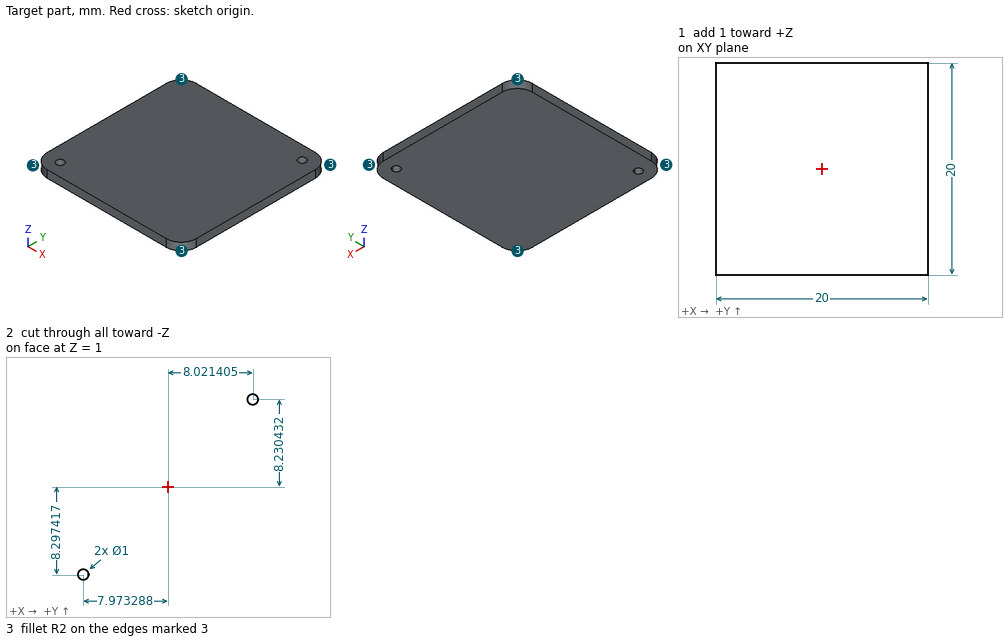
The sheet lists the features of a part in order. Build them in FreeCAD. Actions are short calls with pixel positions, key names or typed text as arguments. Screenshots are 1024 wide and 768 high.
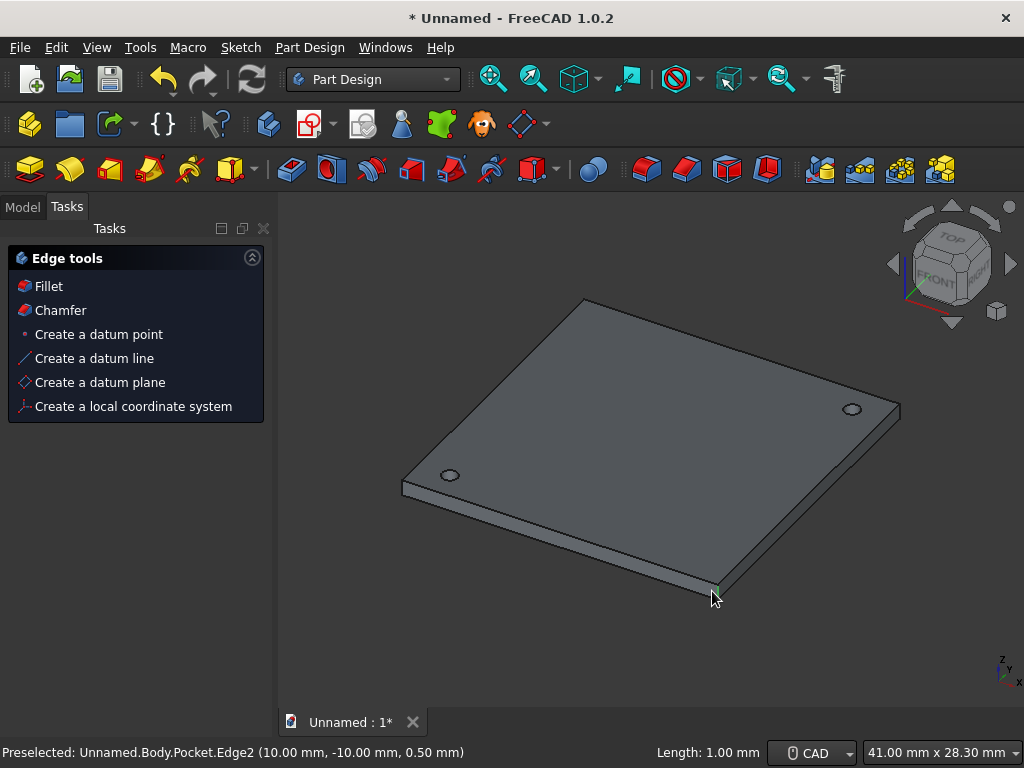
scroll(402, 487, up, 4)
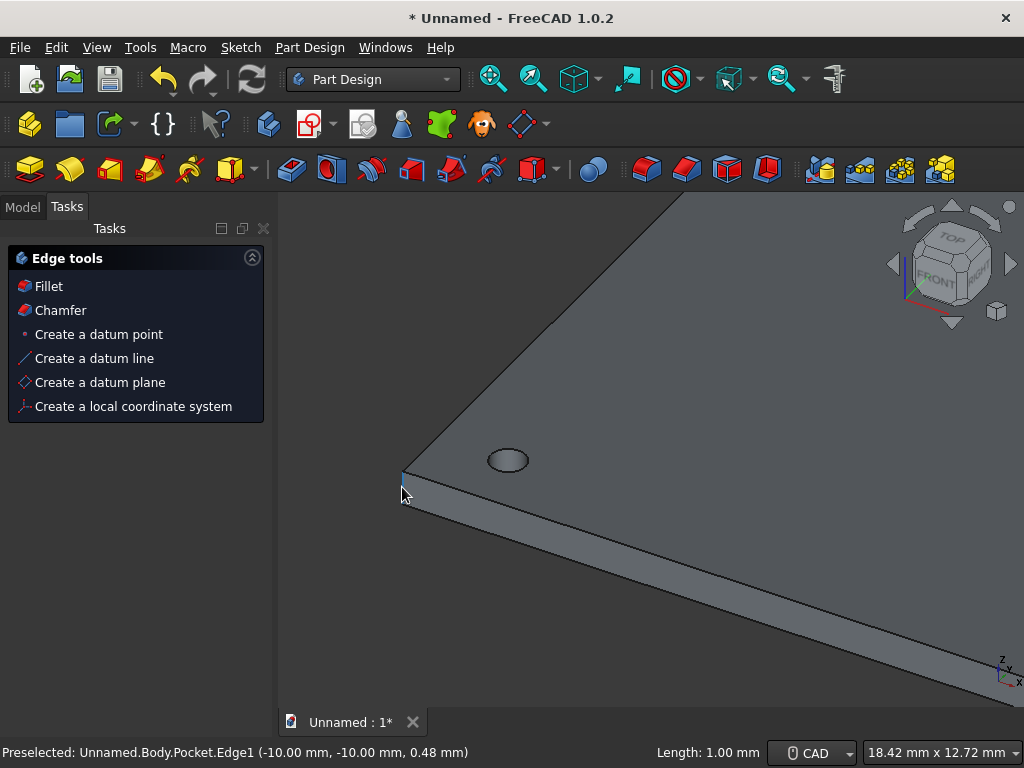
key(v)
key(f)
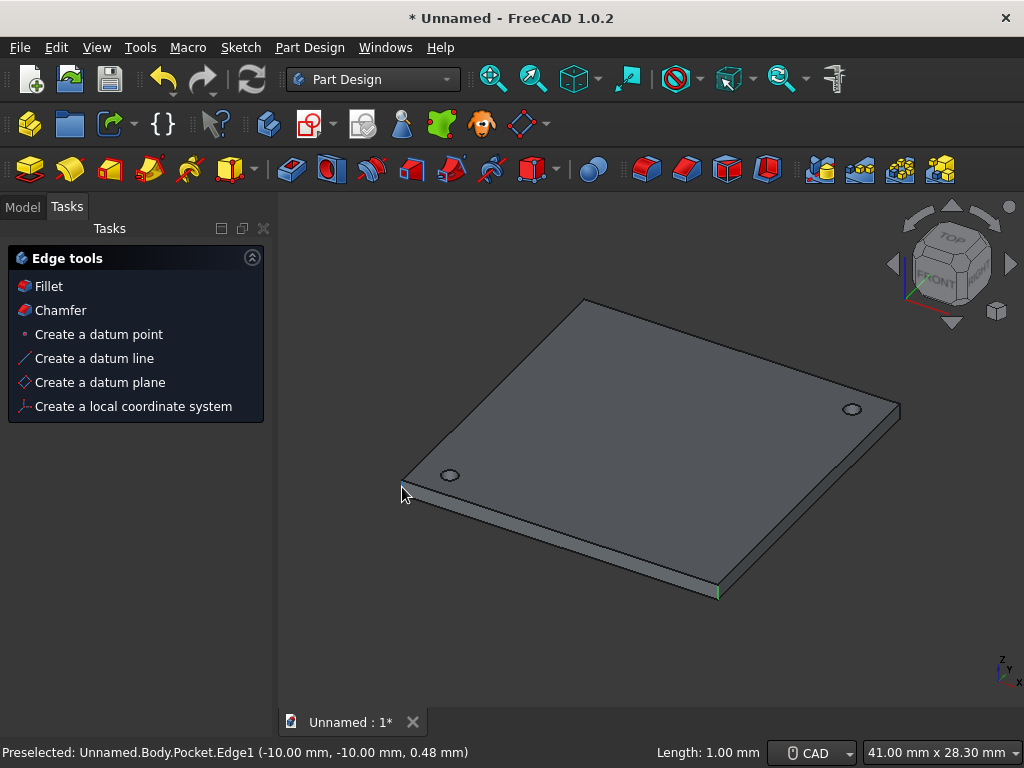
key(0)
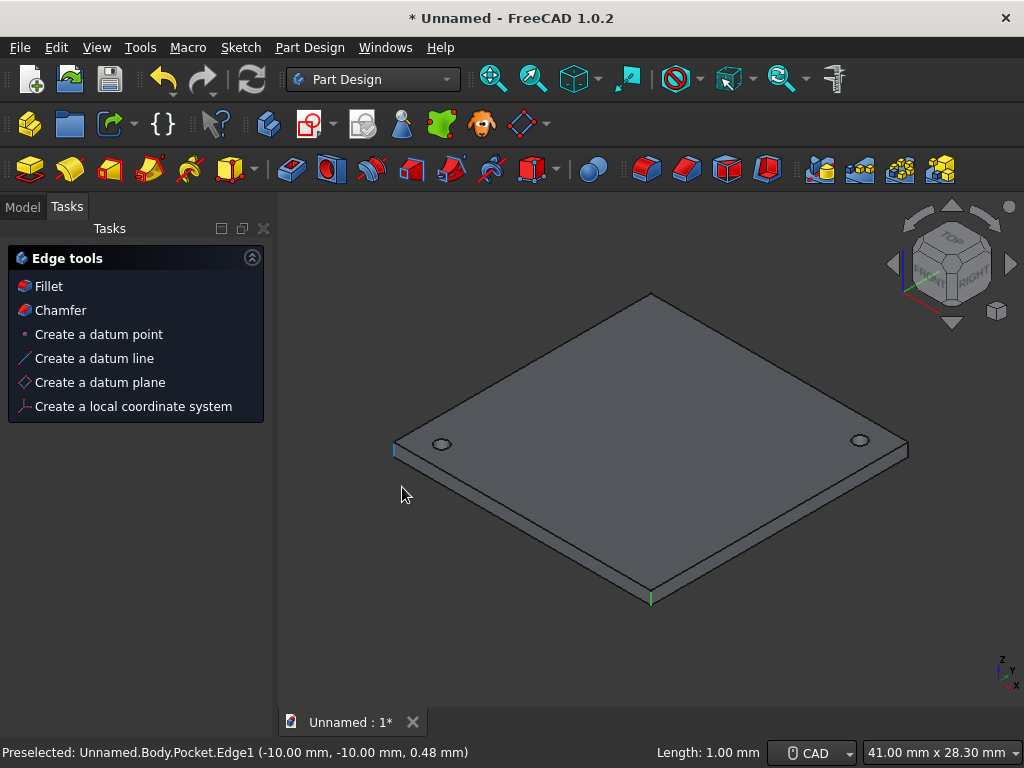
scroll(394, 449, up, 4)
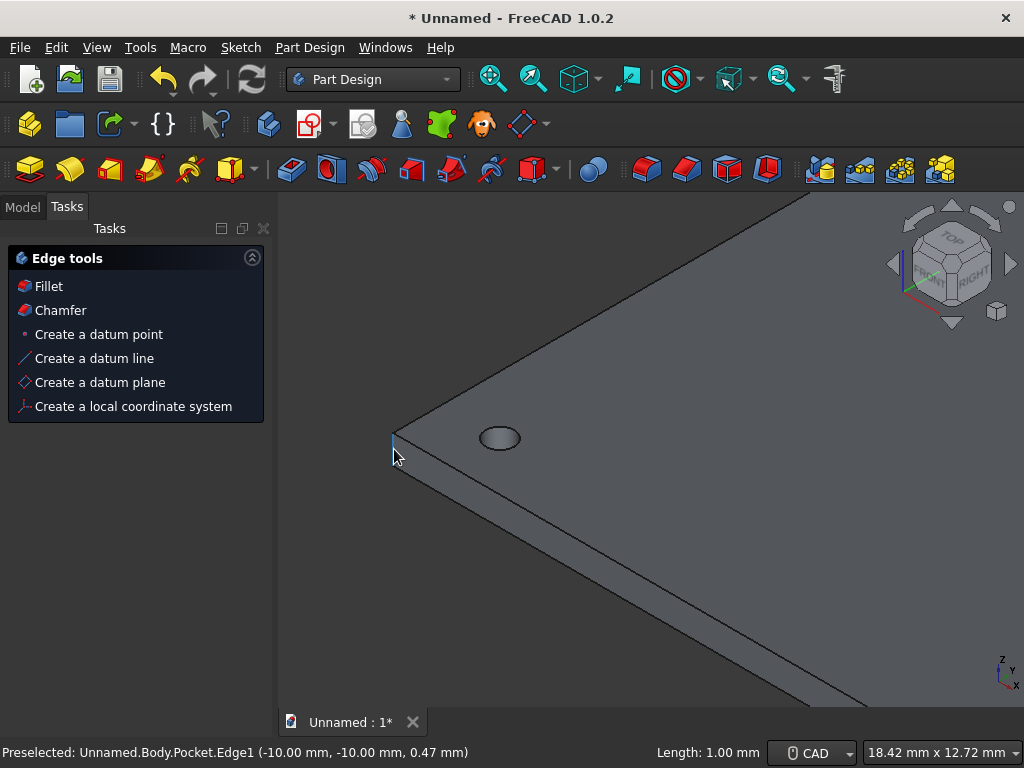
key(v)
key(f)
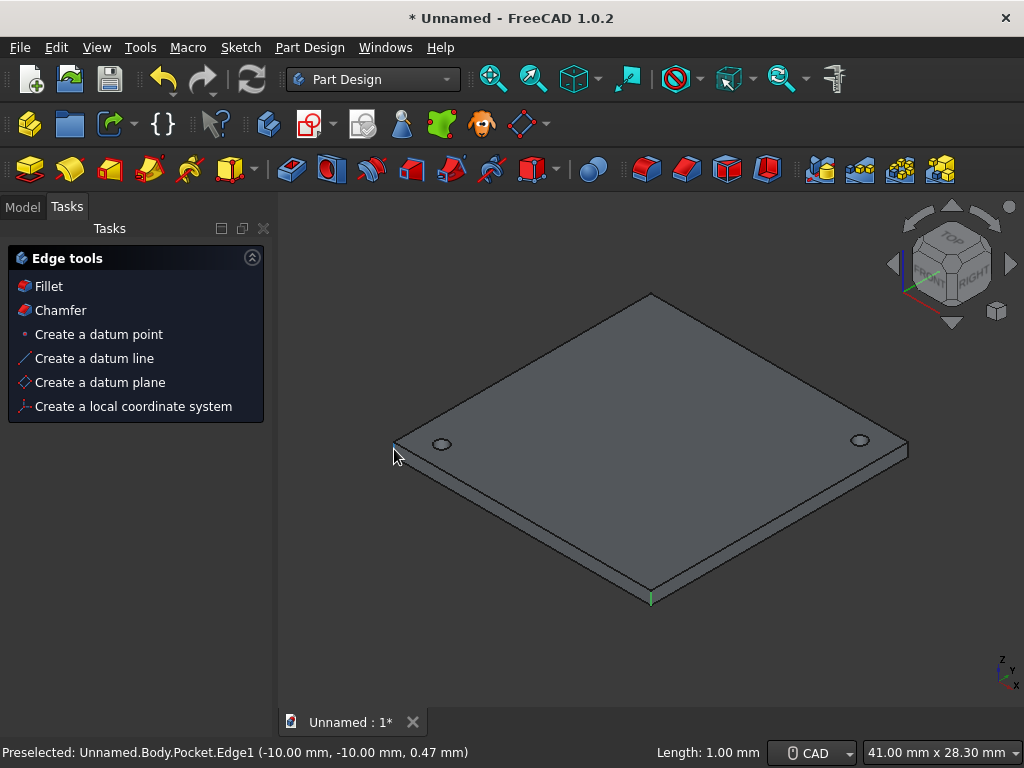
key(2)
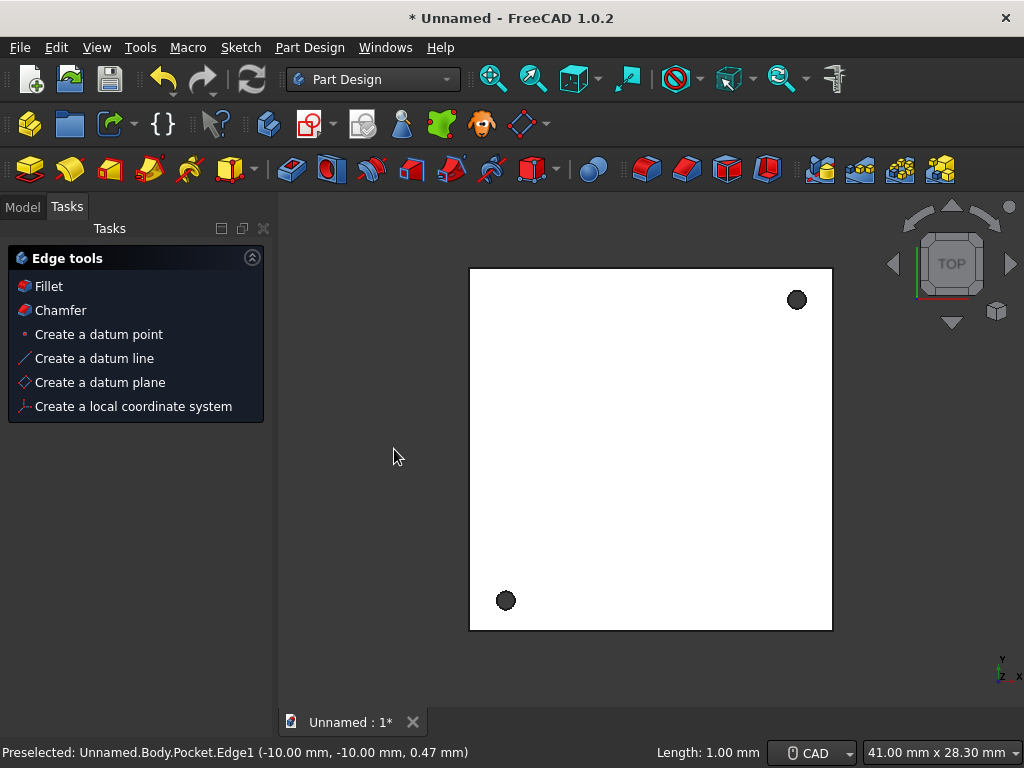
scroll(469, 630, up, 4)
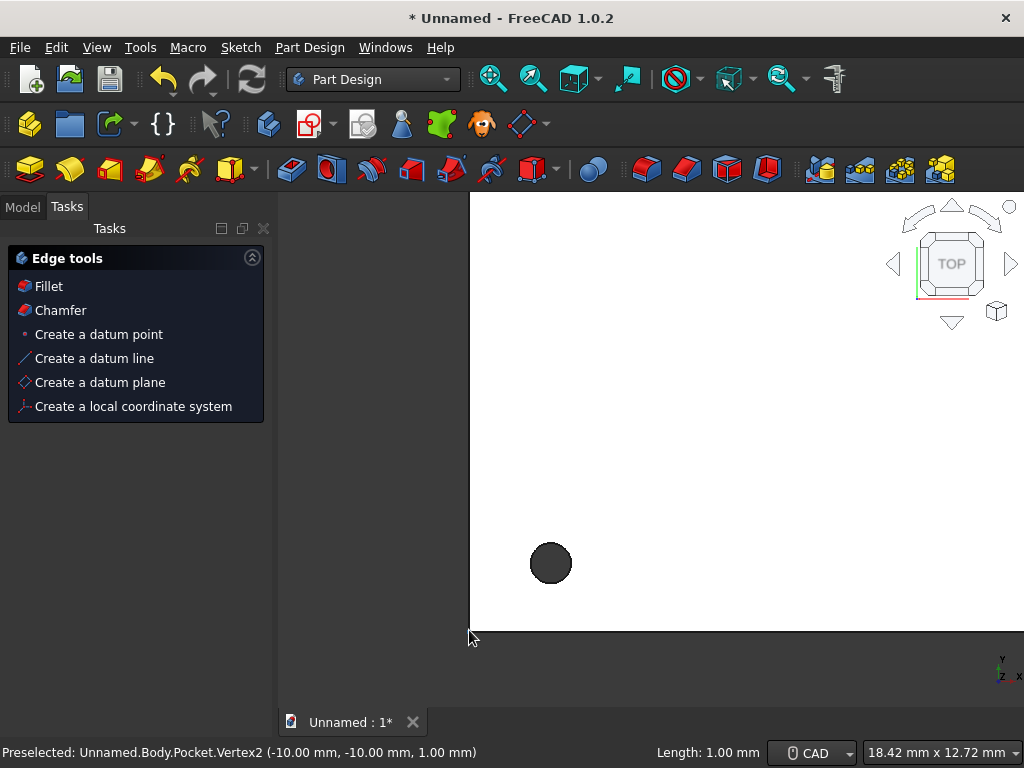
click(494, 80)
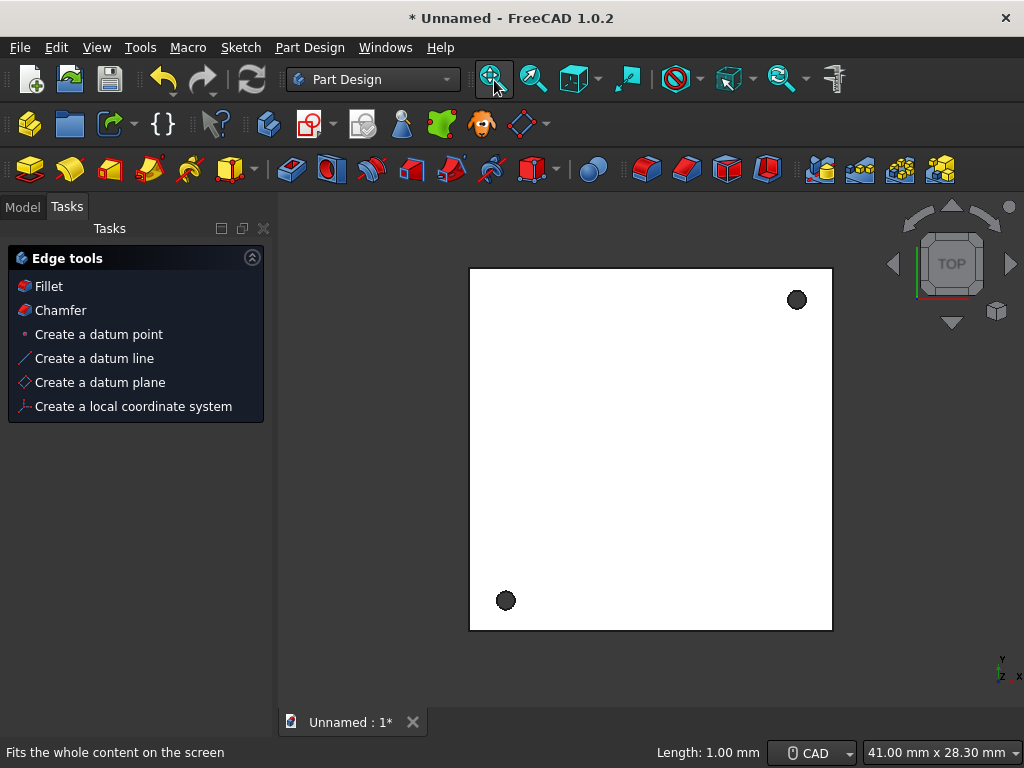
key(1)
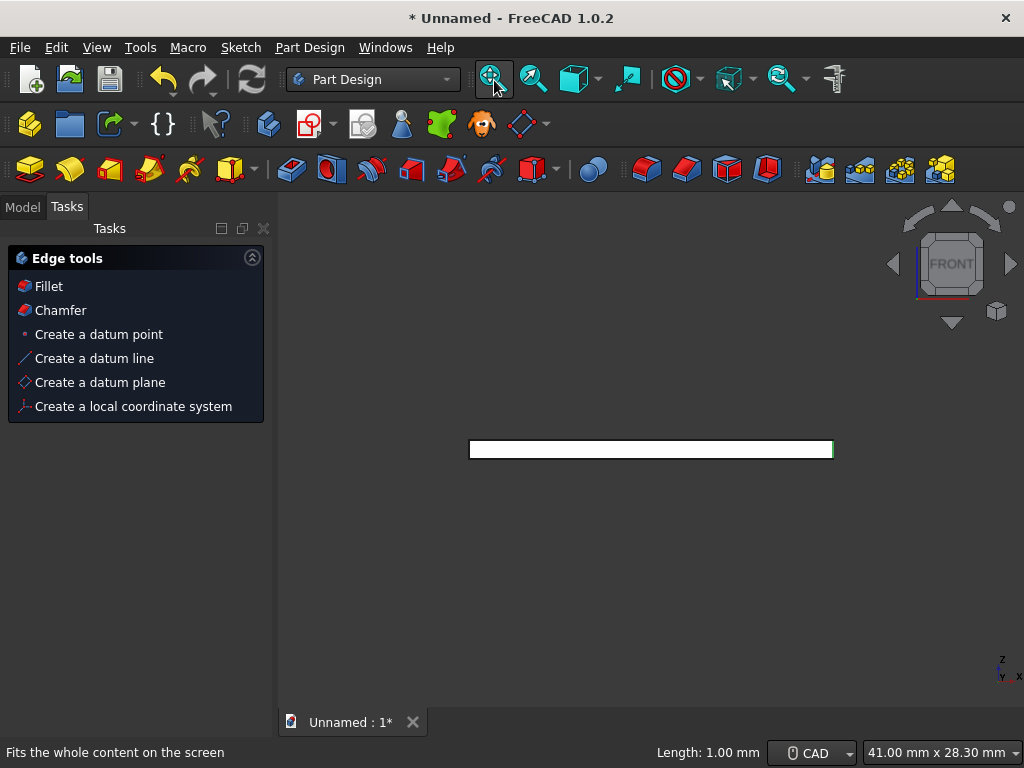
click(469, 449, ctrl)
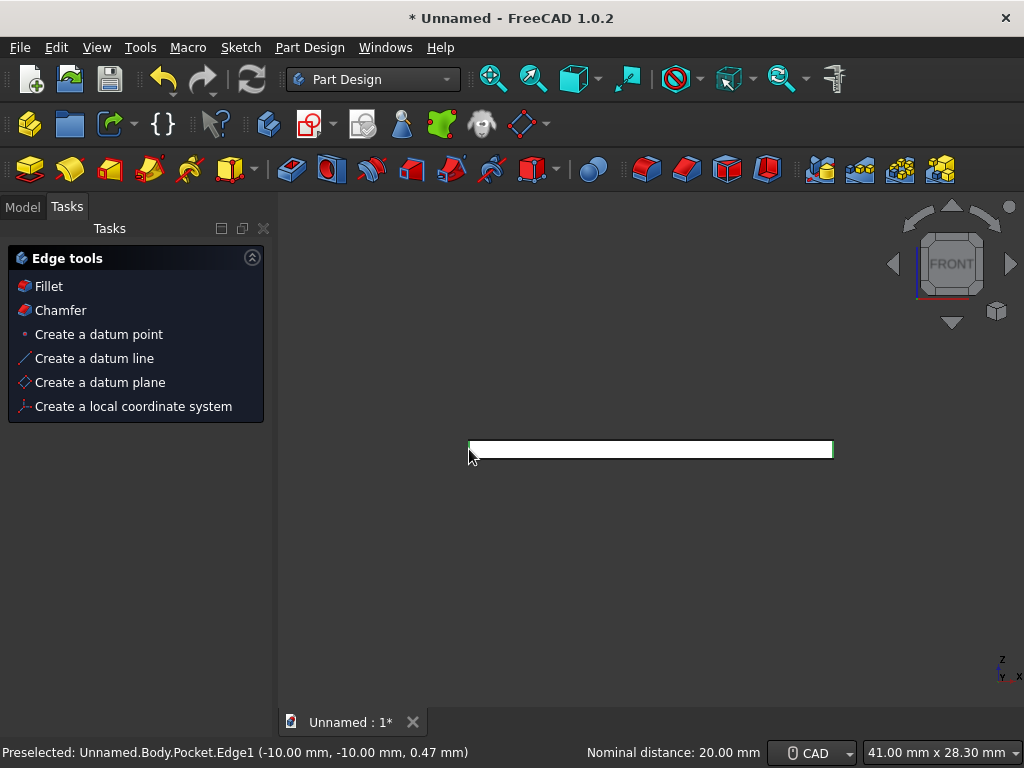
scroll(469, 449, up, 4)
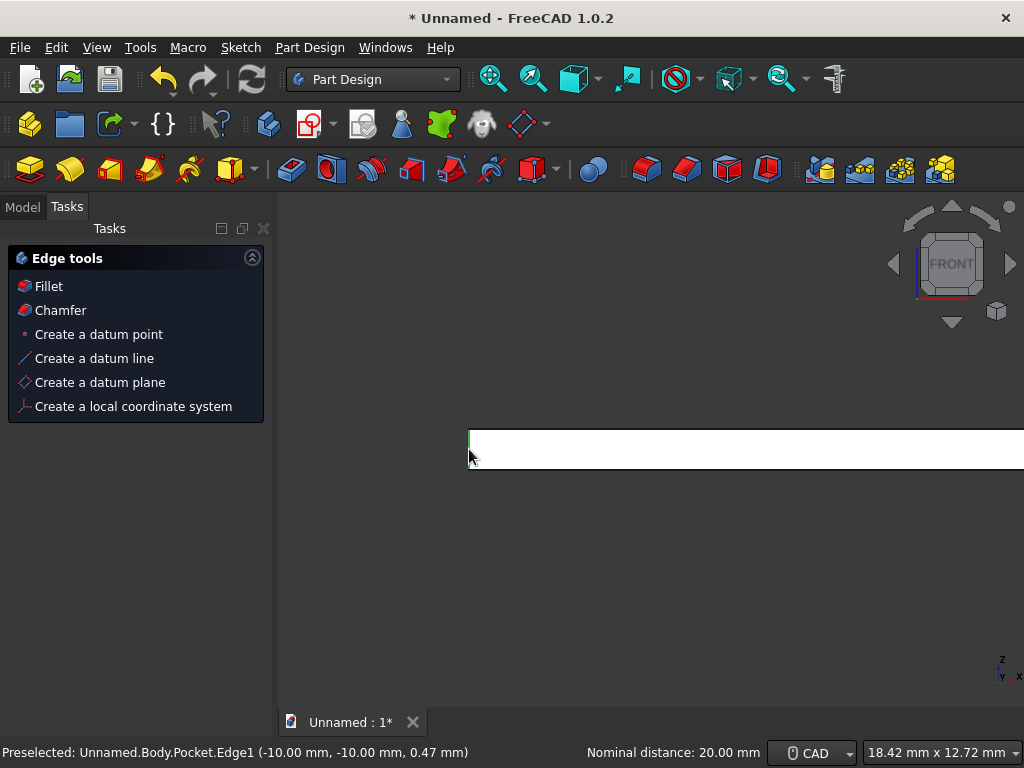
key(v)
key(f)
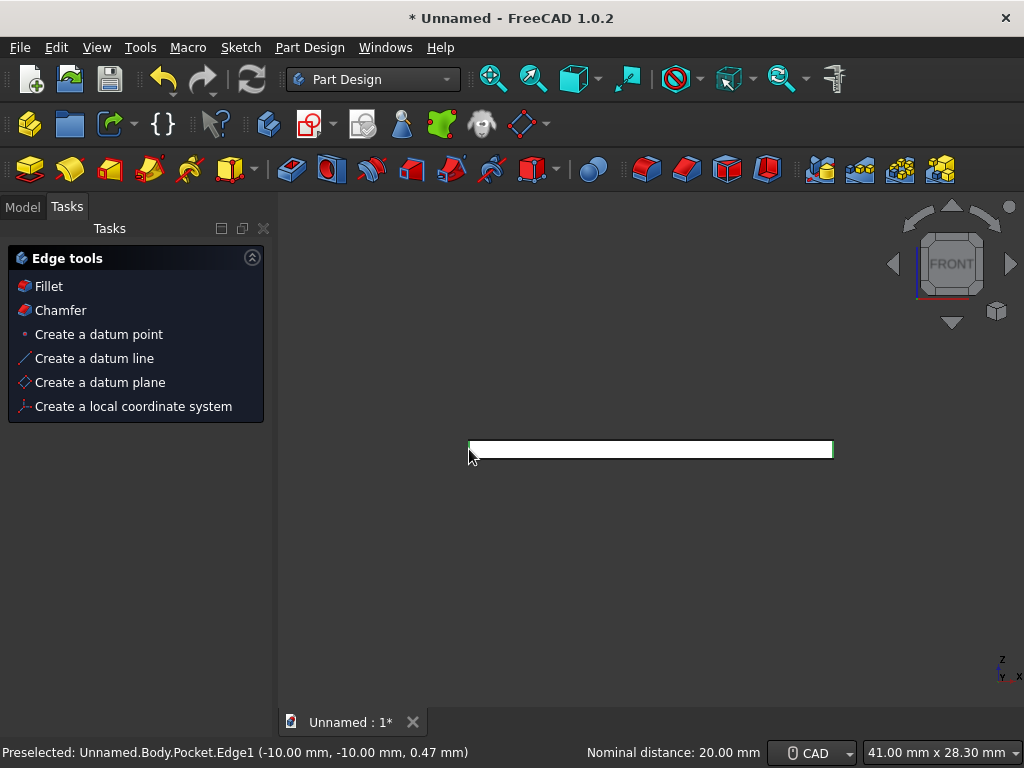
key(3)